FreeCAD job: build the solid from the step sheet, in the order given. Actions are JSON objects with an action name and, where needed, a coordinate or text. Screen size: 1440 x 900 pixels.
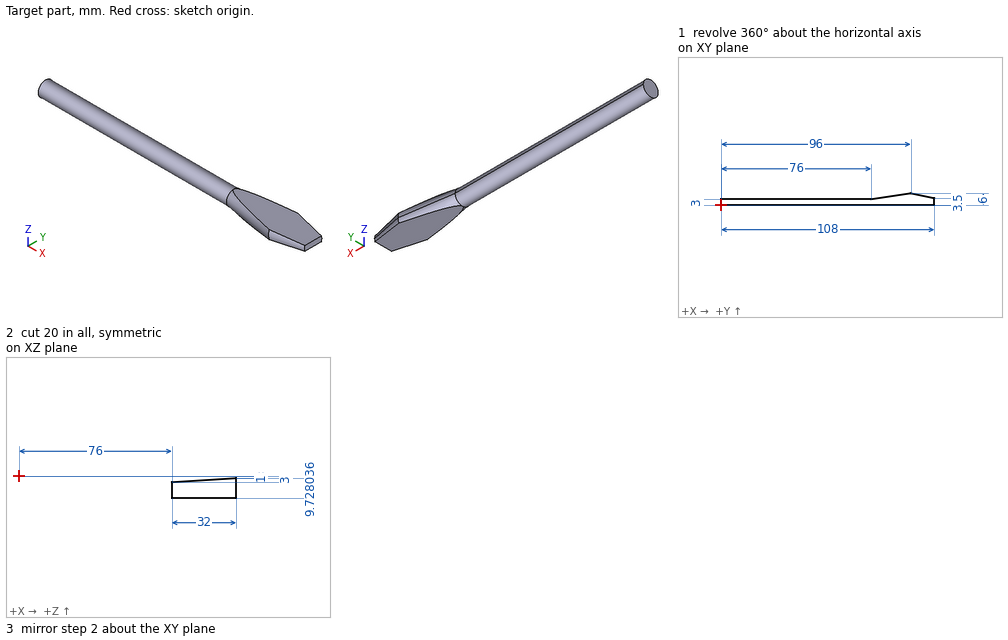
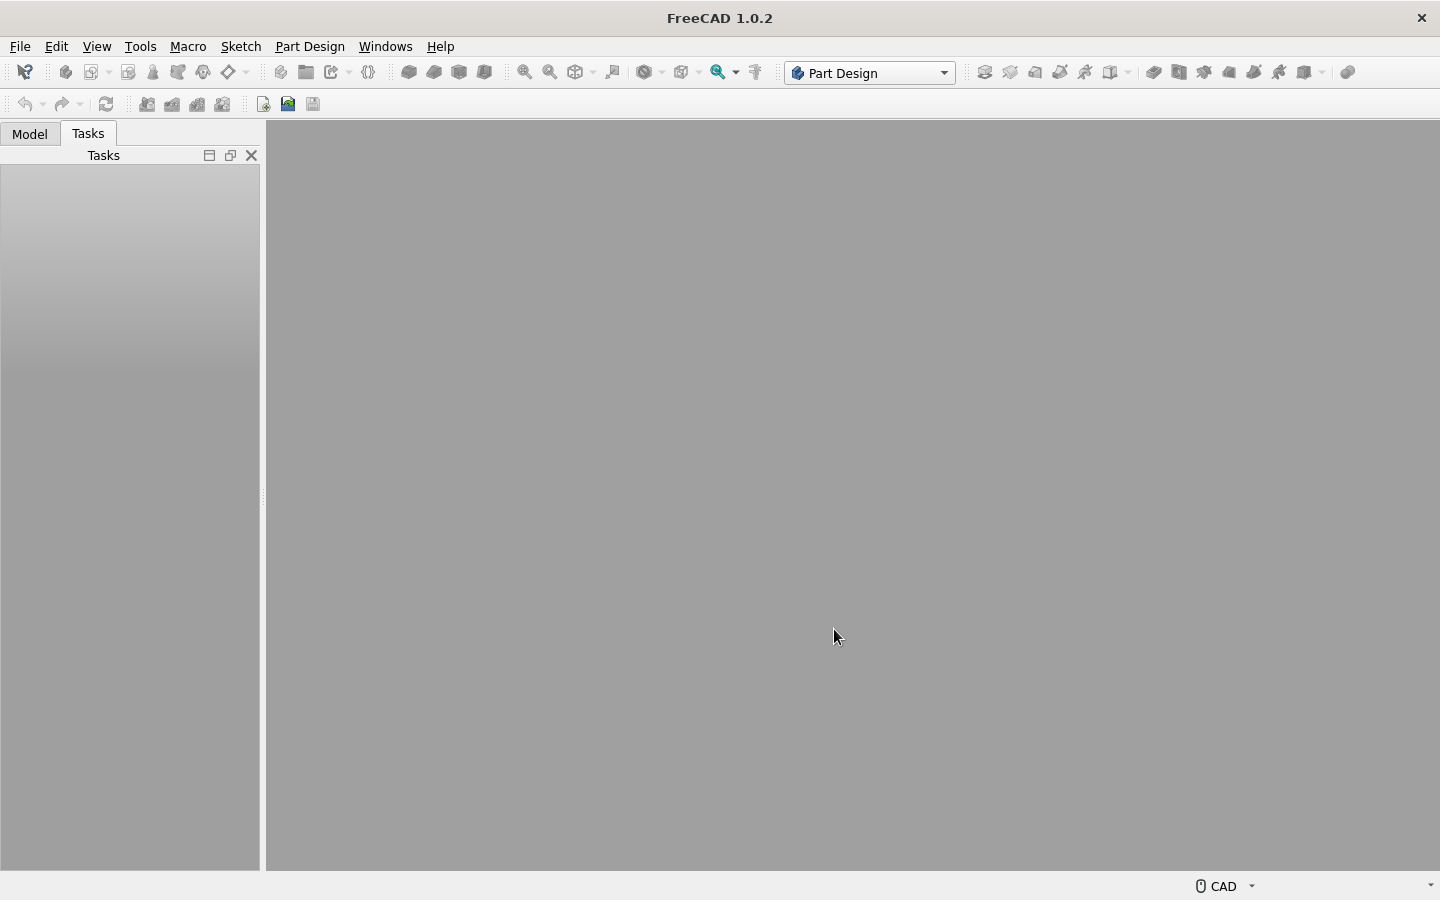
{"action": "key", "text": "ctrl+n"}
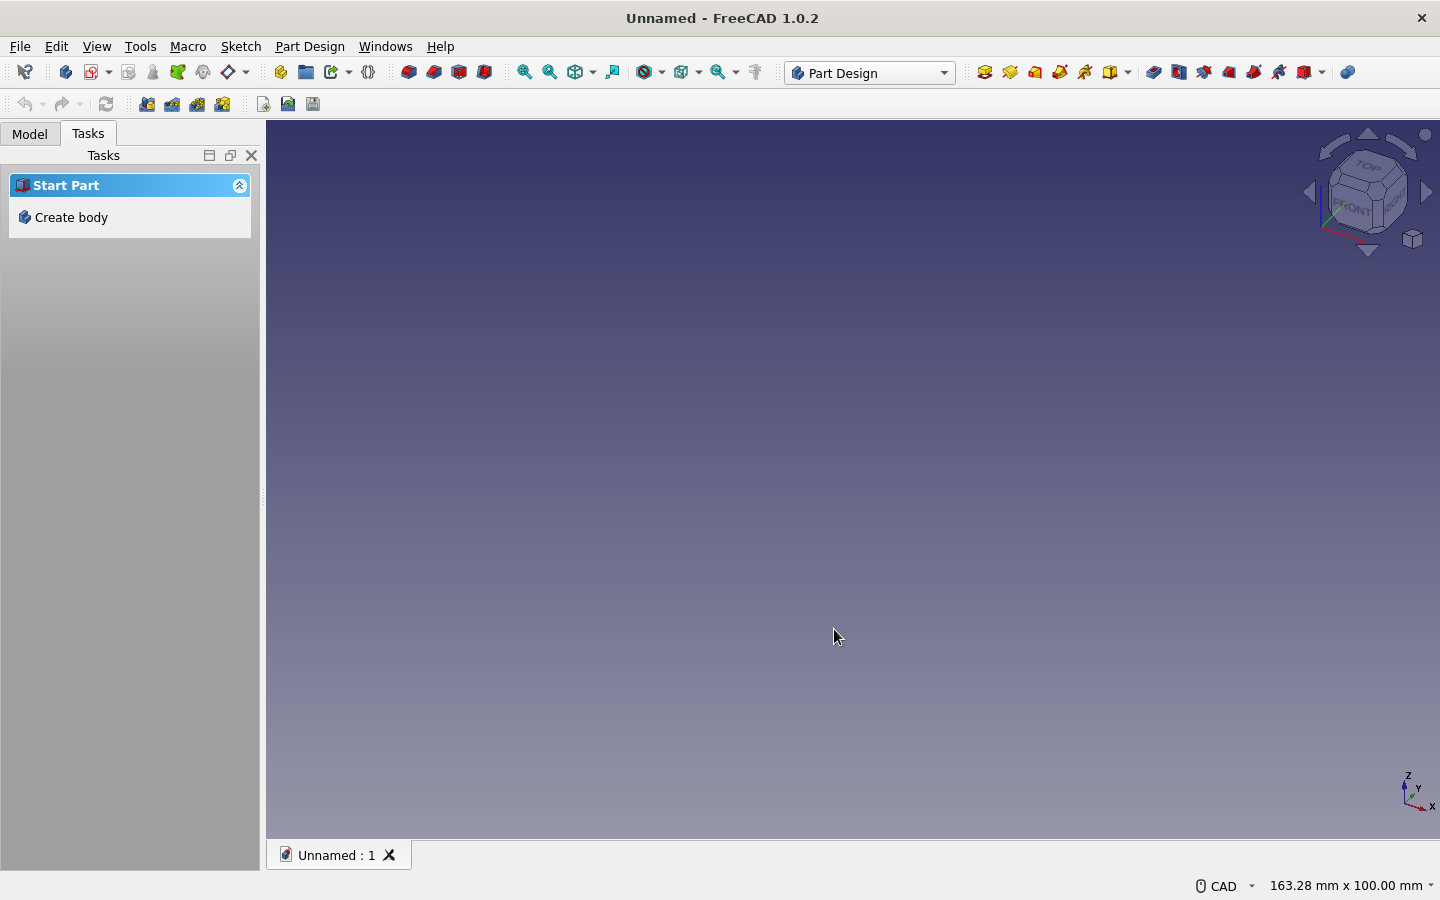
{"action": "left_click", "coordinate": [90, 72]}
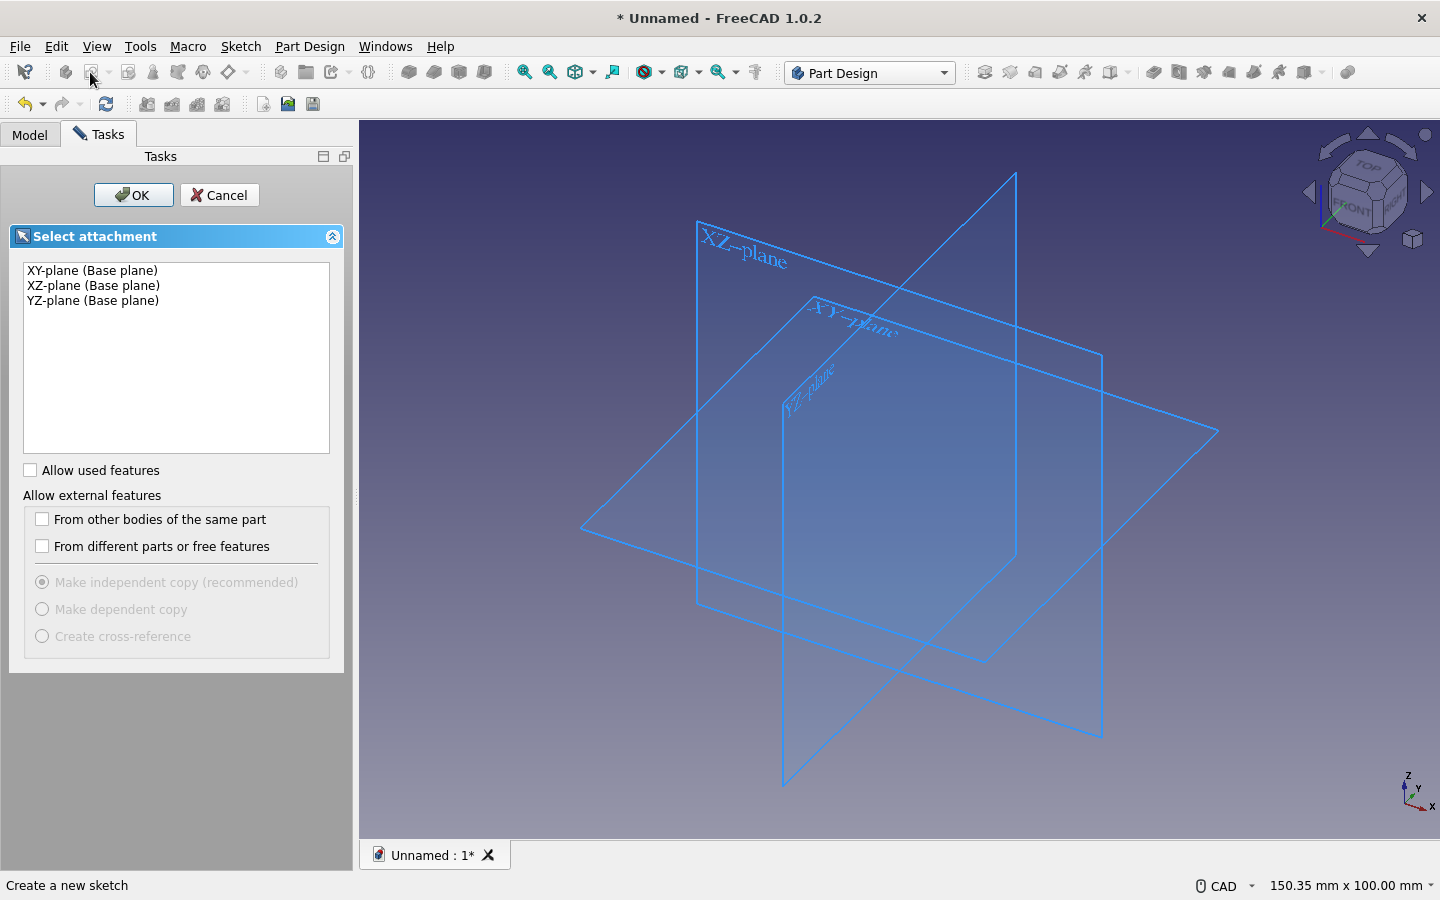
{"action": "left_click", "coordinate": [84, 270]}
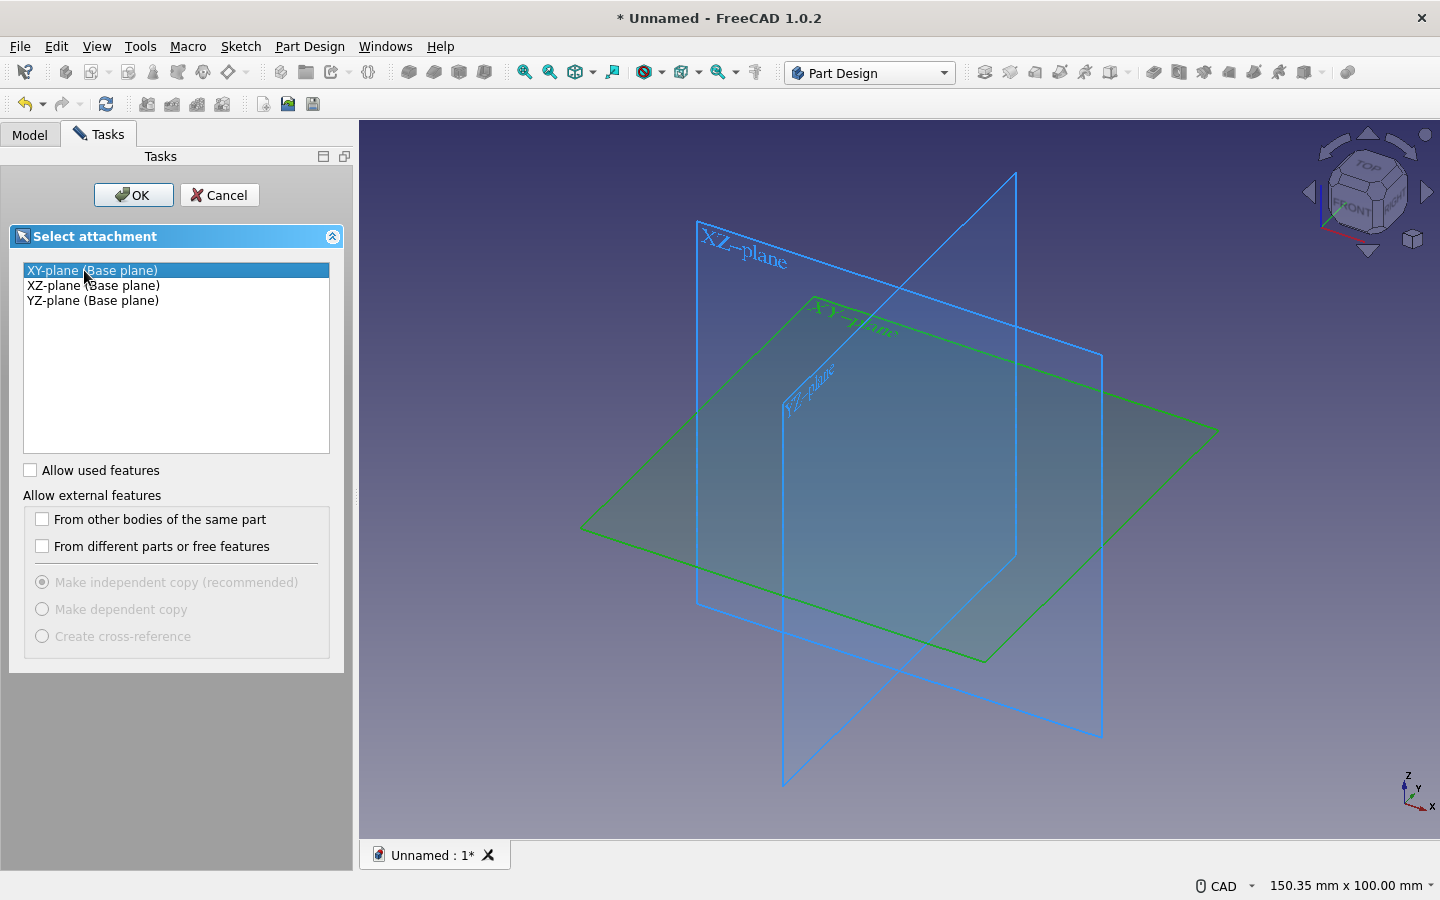
{"action": "left_click", "coordinate": [134, 195]}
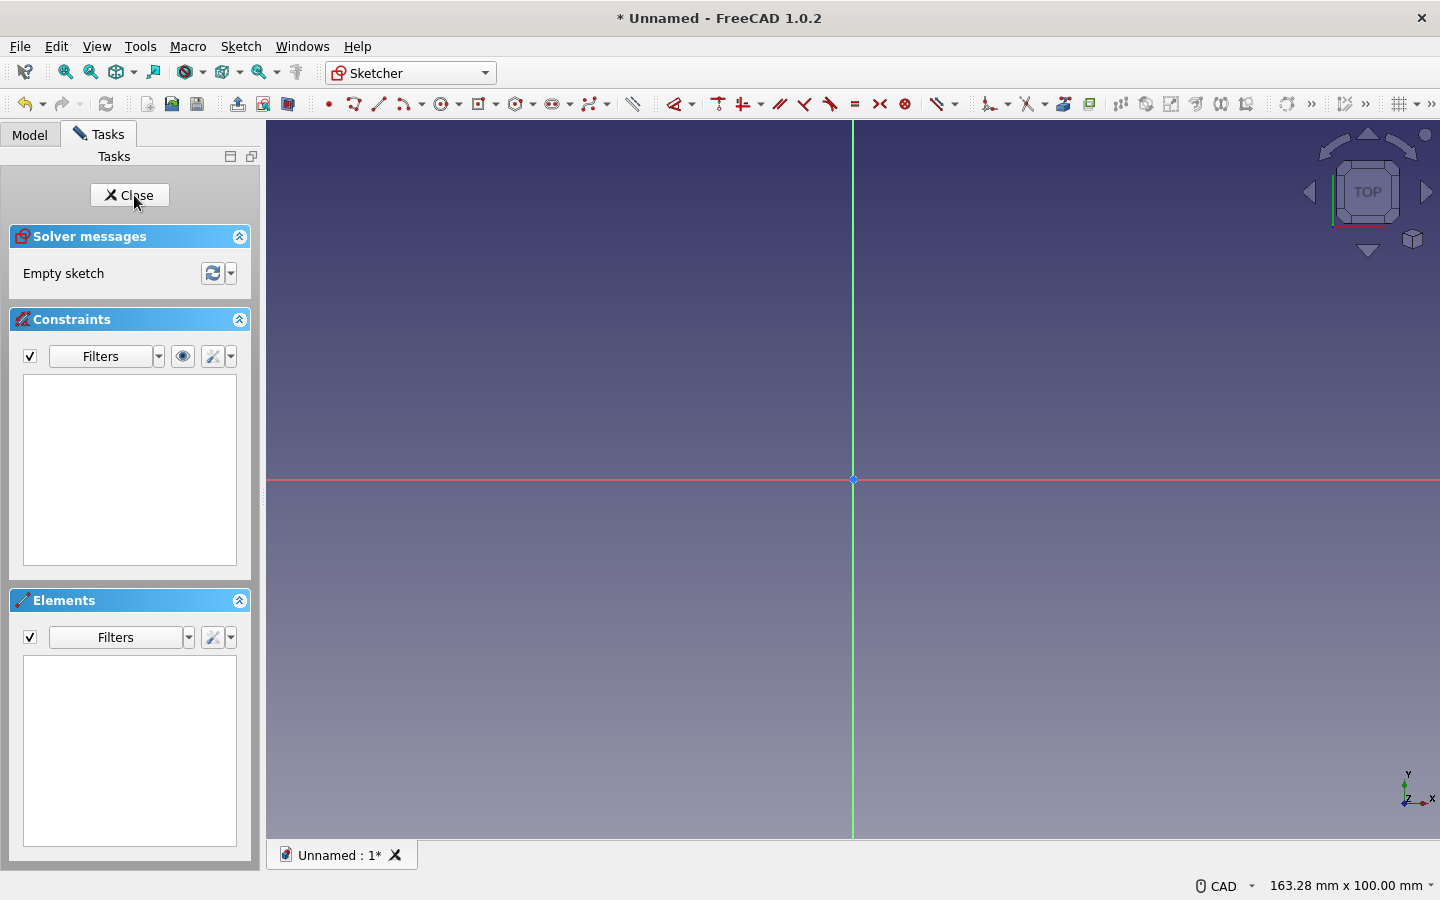
{"action": "scroll", "coordinate": [294, 523], "scroll_direction": "down", "scroll_amount": 2}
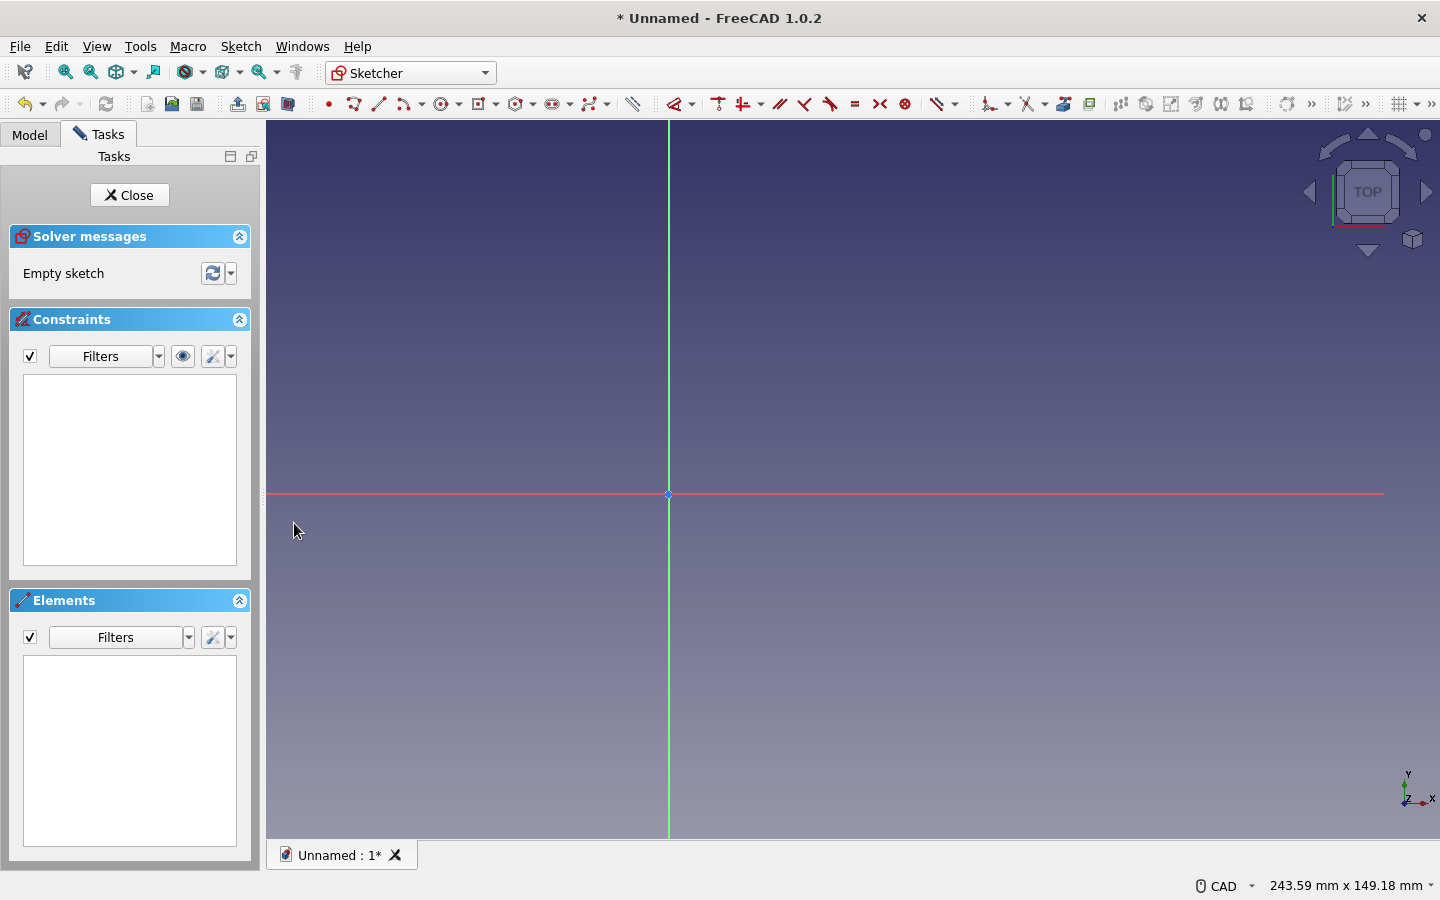
{"action": "left_click", "coordinate": [354, 104]}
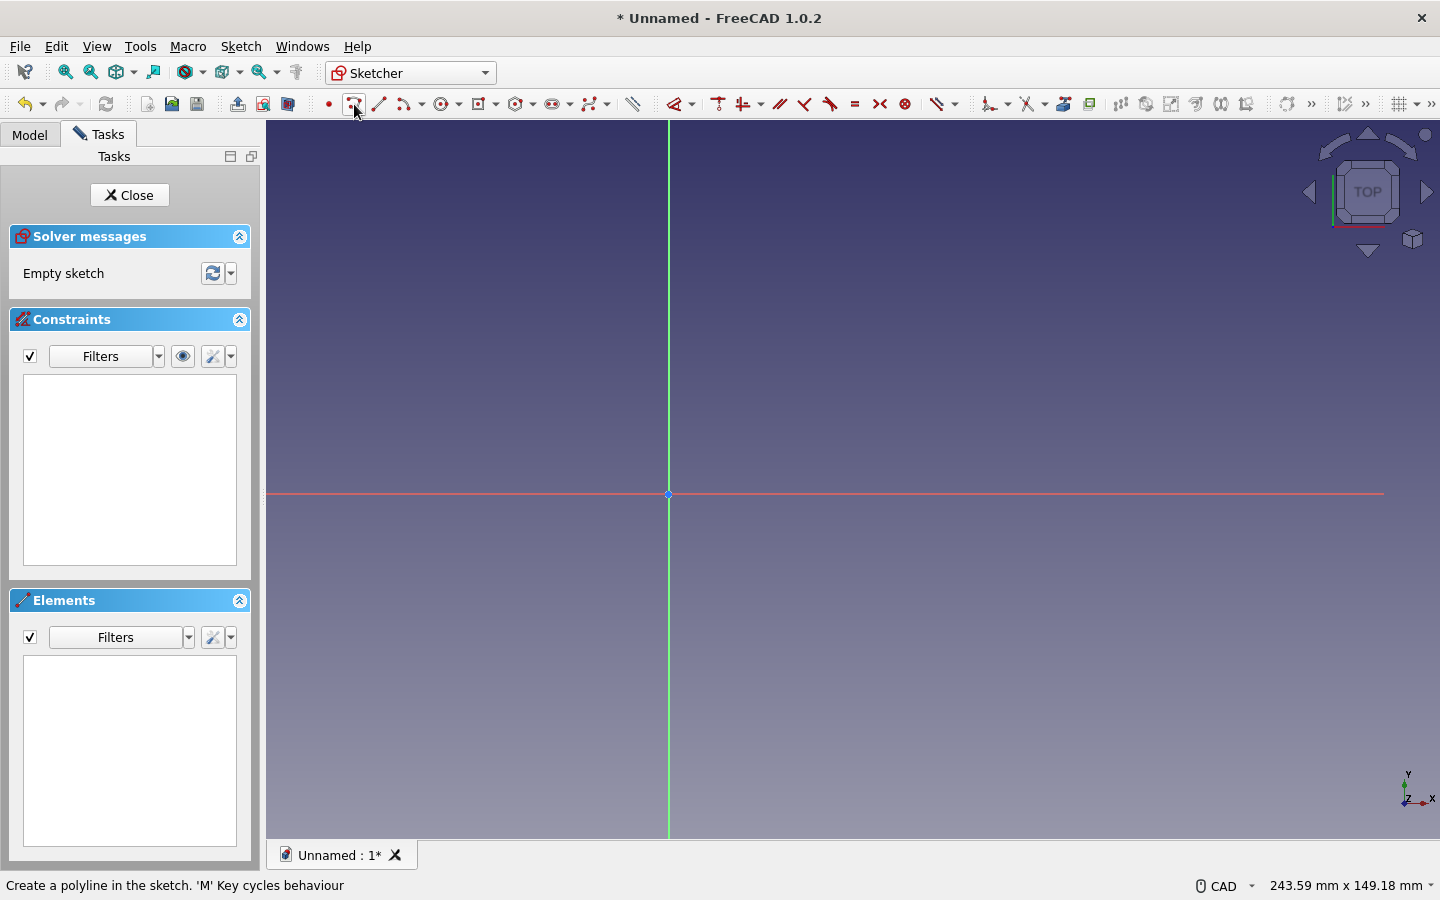
{"action": "left_click", "coordinate": [669, 494]}
{"action": "left_click", "coordinate": [1189, 485]}
{"action": "left_click", "coordinate": [1189, 477]}
{"action": "left_click", "coordinate": [1131, 465]}
{"action": "left_click", "coordinate": [1035, 480]}
{"action": "left_click", "coordinate": [678, 480]}
{"action": "left_click", "coordinate": [669, 494]}
{"action": "key", "text": "Escape"}
{"action": "key", "text": "Escape"}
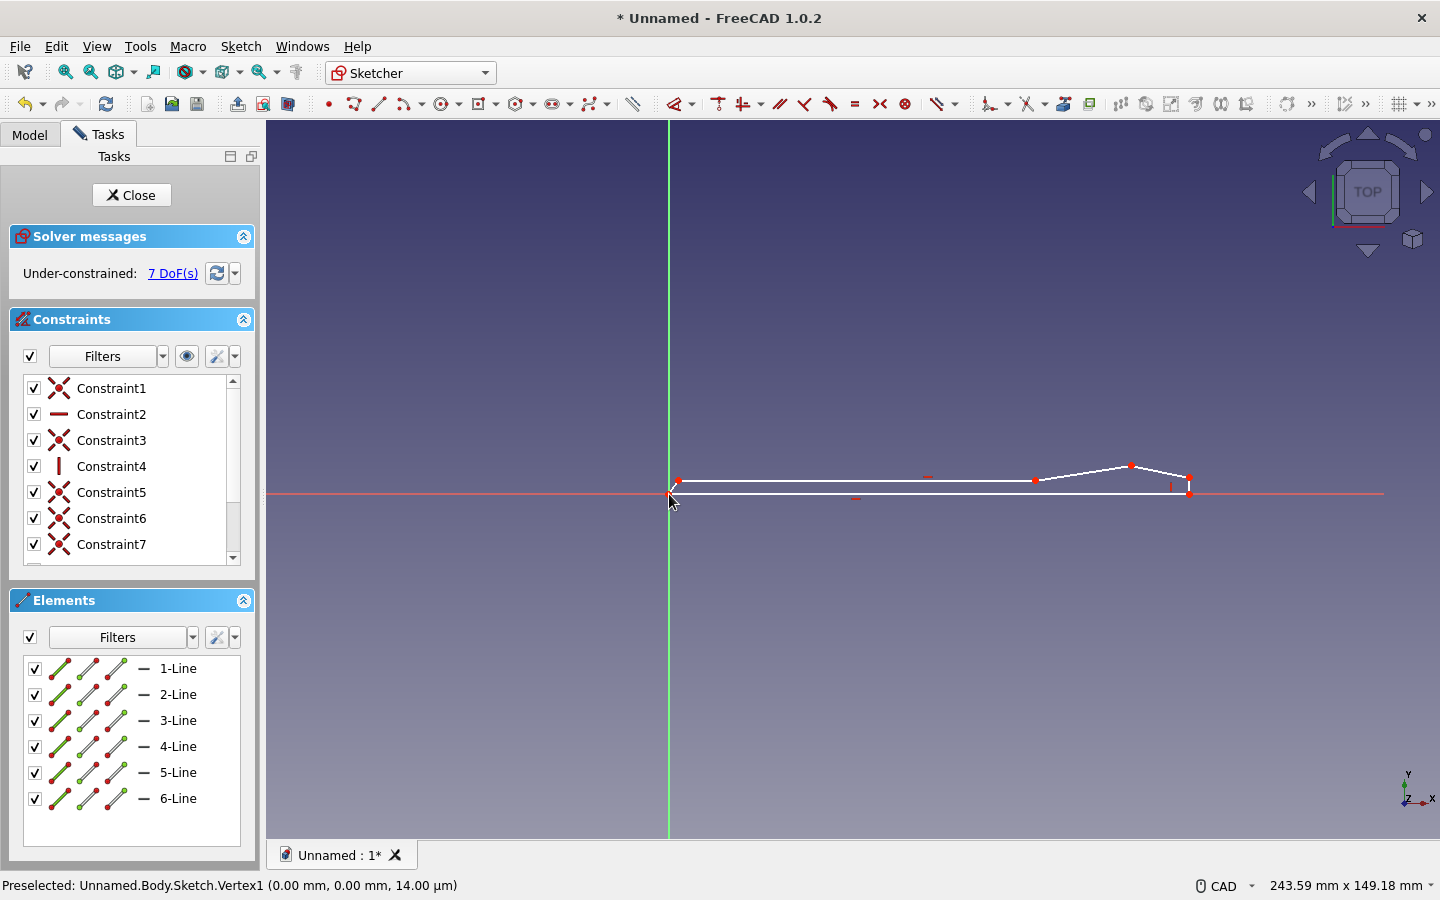
{"action": "scroll", "coordinate": [674, 486], "scroll_direction": "up", "scroll_amount": 5}